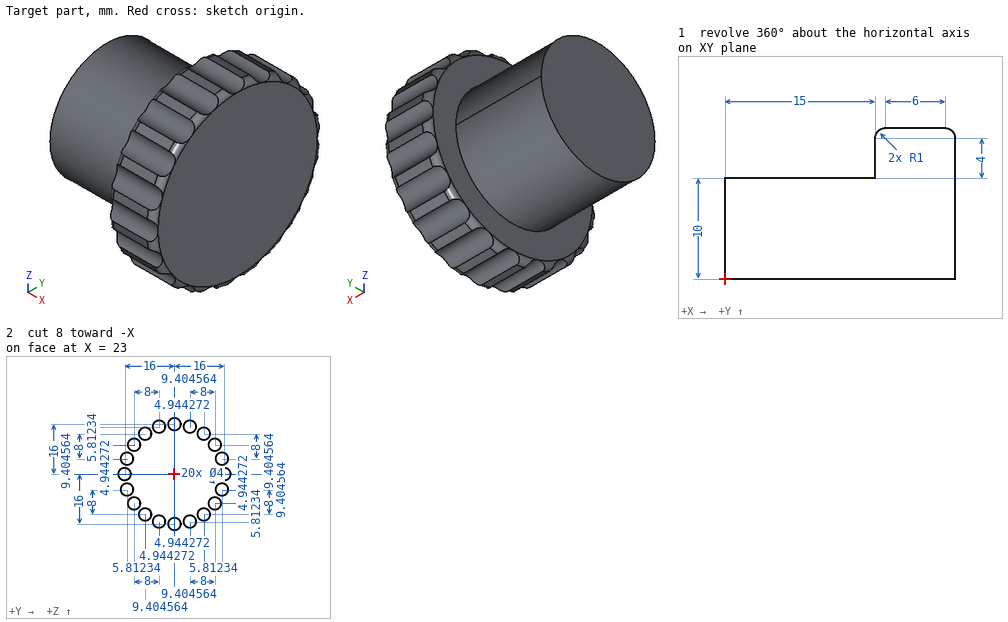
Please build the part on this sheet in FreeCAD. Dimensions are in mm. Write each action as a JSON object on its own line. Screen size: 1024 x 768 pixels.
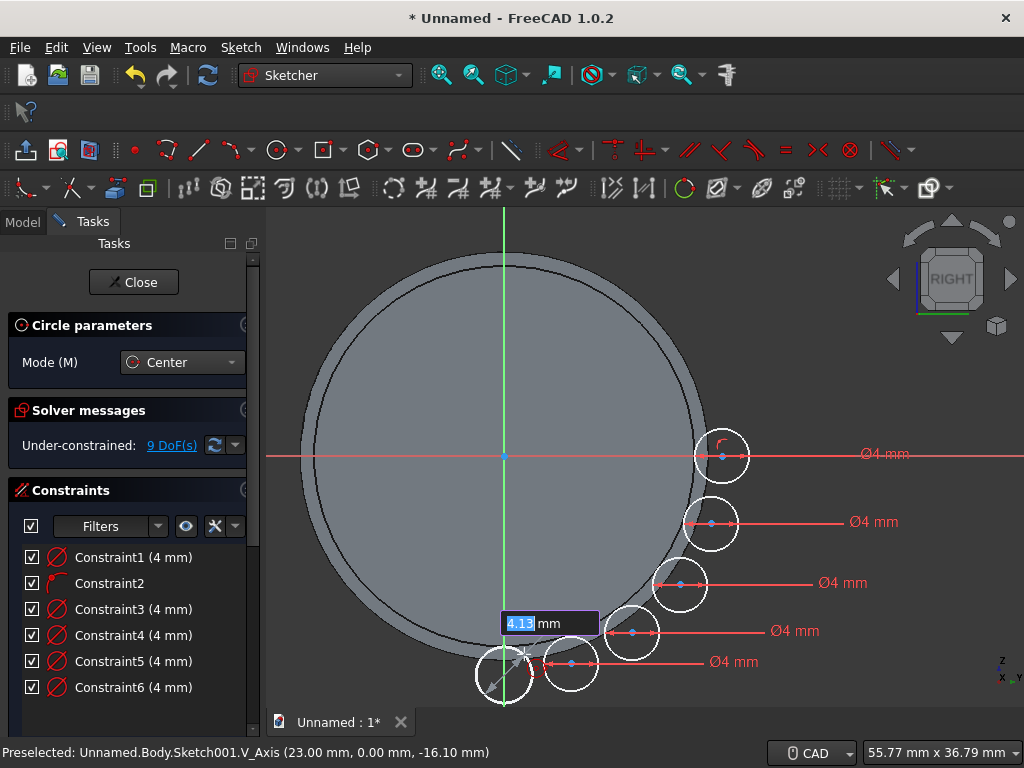
{"action": "type", "text": "4"}
{"action": "key", "text": "Return"}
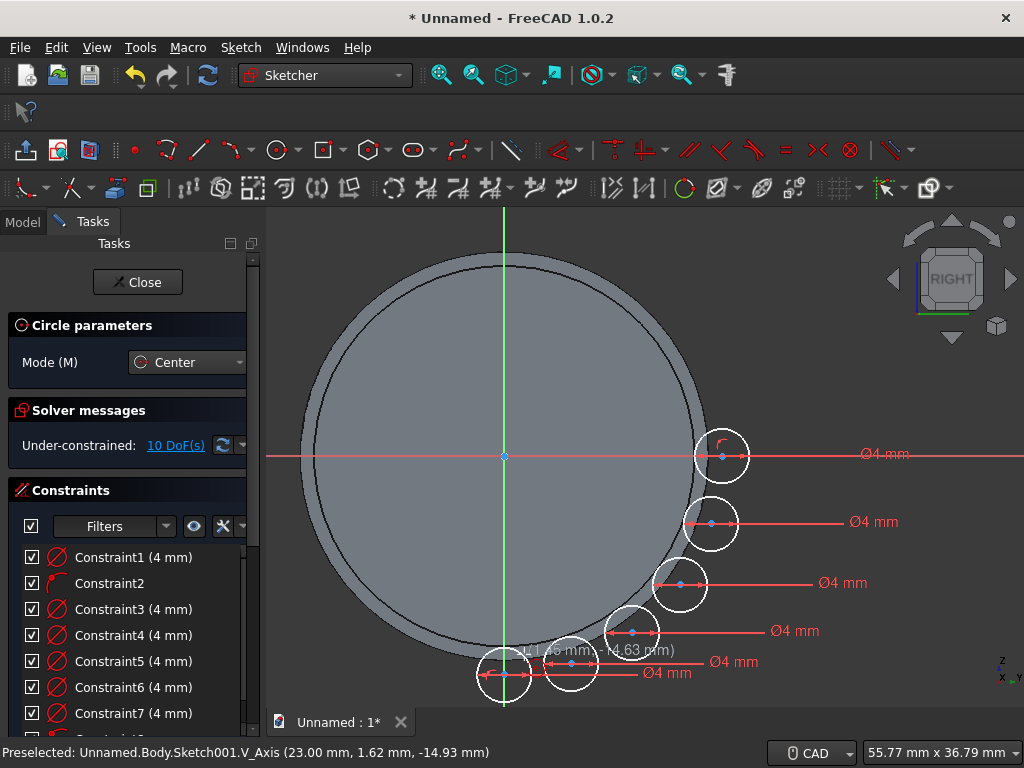
{"action": "left_click", "coordinate": [437, 663]}
{"action": "mouse_move", "coordinate": [456, 644]}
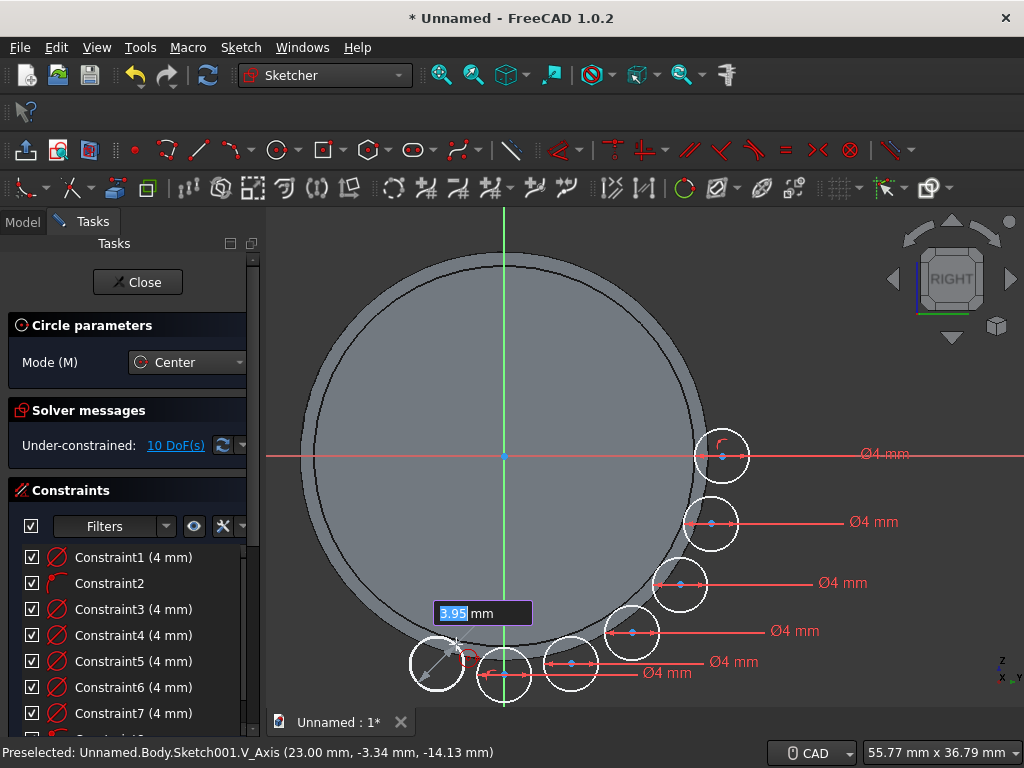
{"action": "type", "text": "4"}
{"action": "key", "text": "Return"}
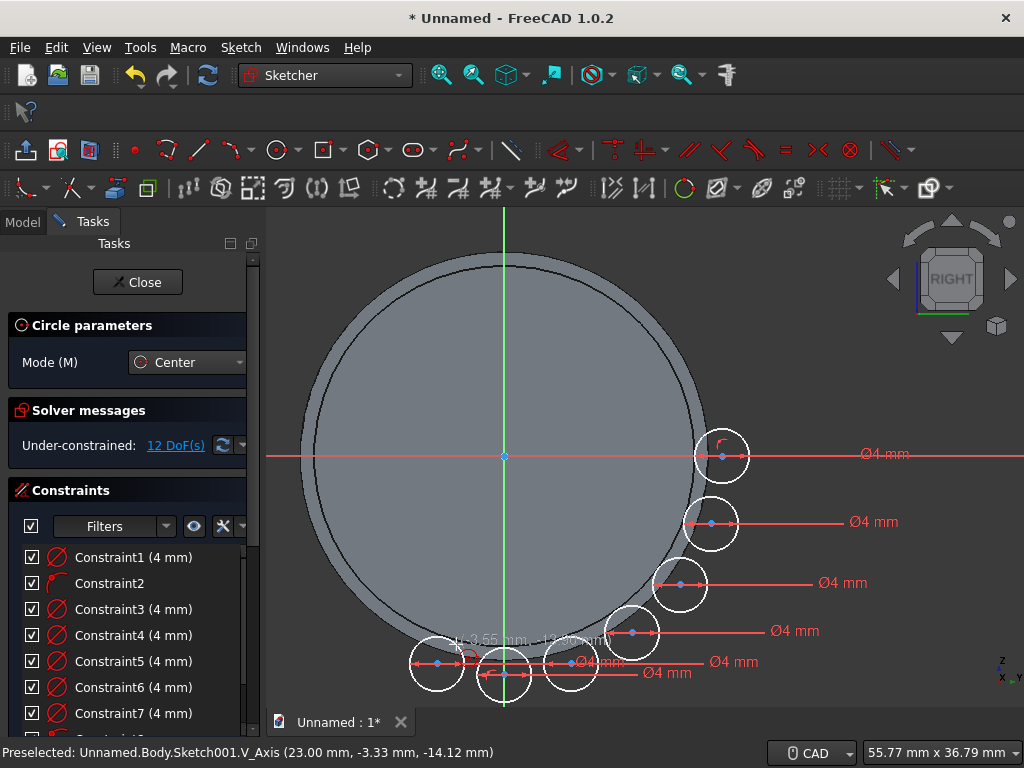
{"action": "left_click", "coordinate": [376, 632]}
{"action": "mouse_move", "coordinate": [396, 613]}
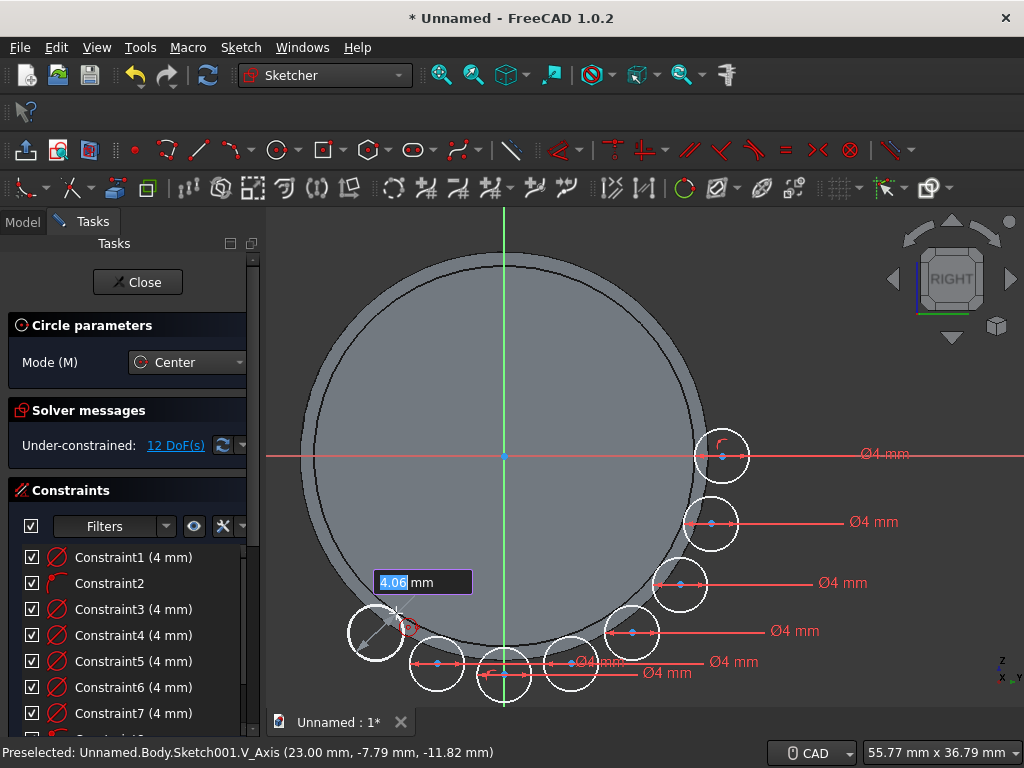
{"action": "type", "text": "4"}
{"action": "key", "text": "Return"}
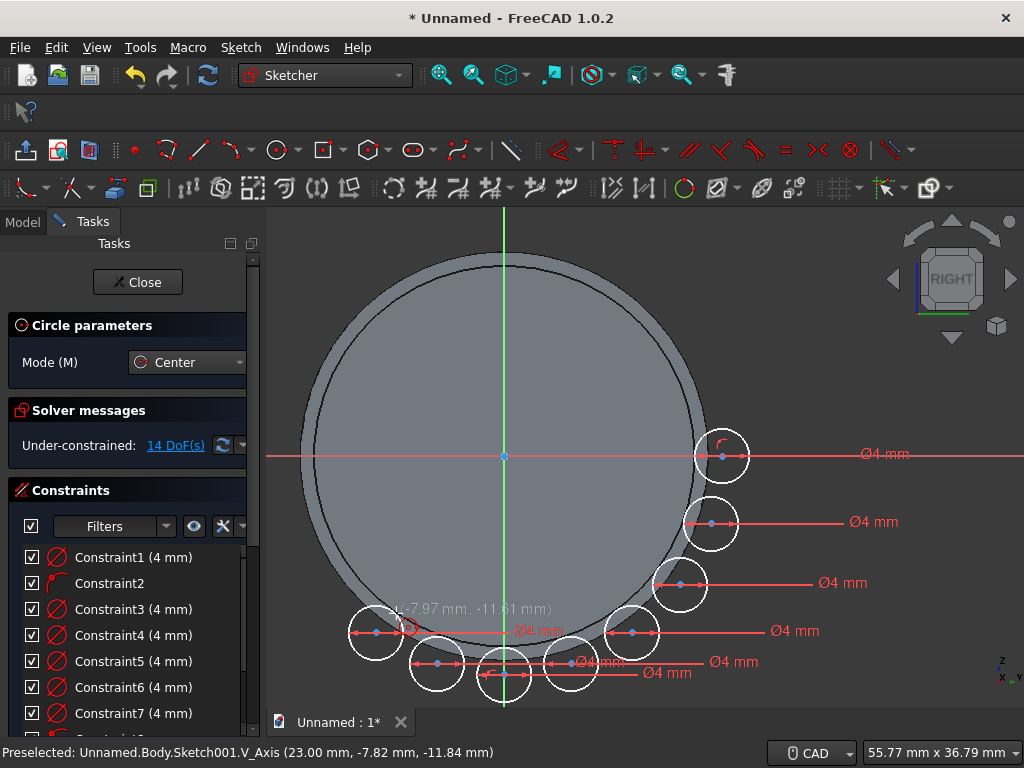
{"action": "left_click", "coordinate": [328, 584]}
{"action": "mouse_move", "coordinate": [348, 565]}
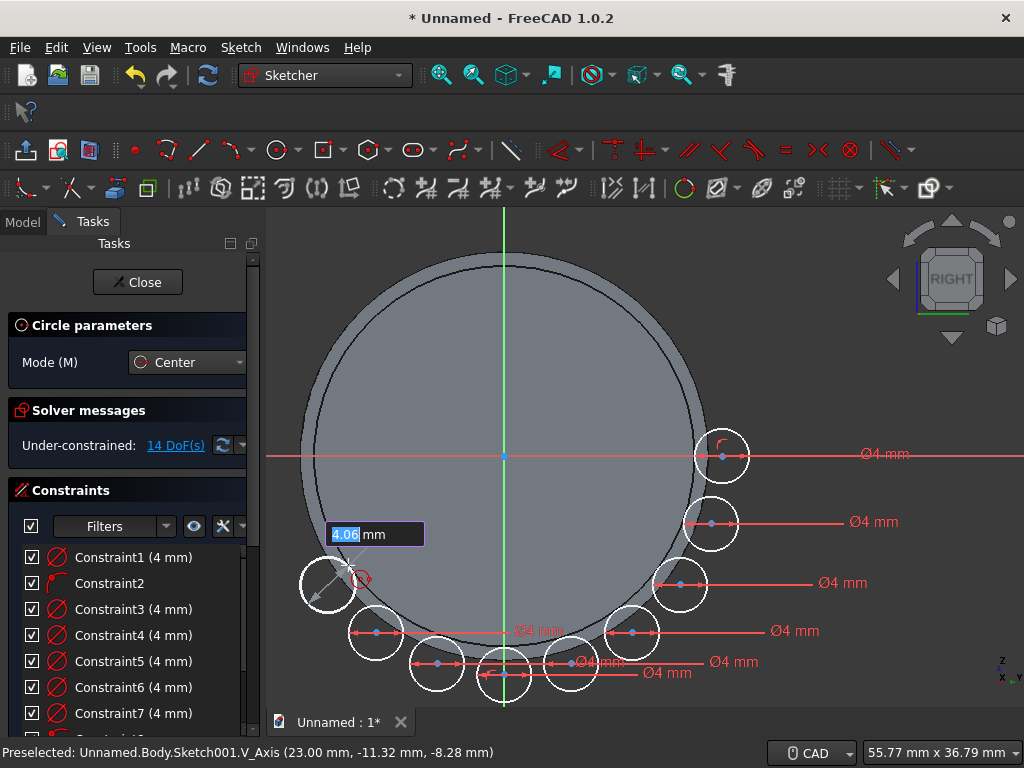
{"action": "type", "text": "4"}
{"action": "key", "text": "Return"}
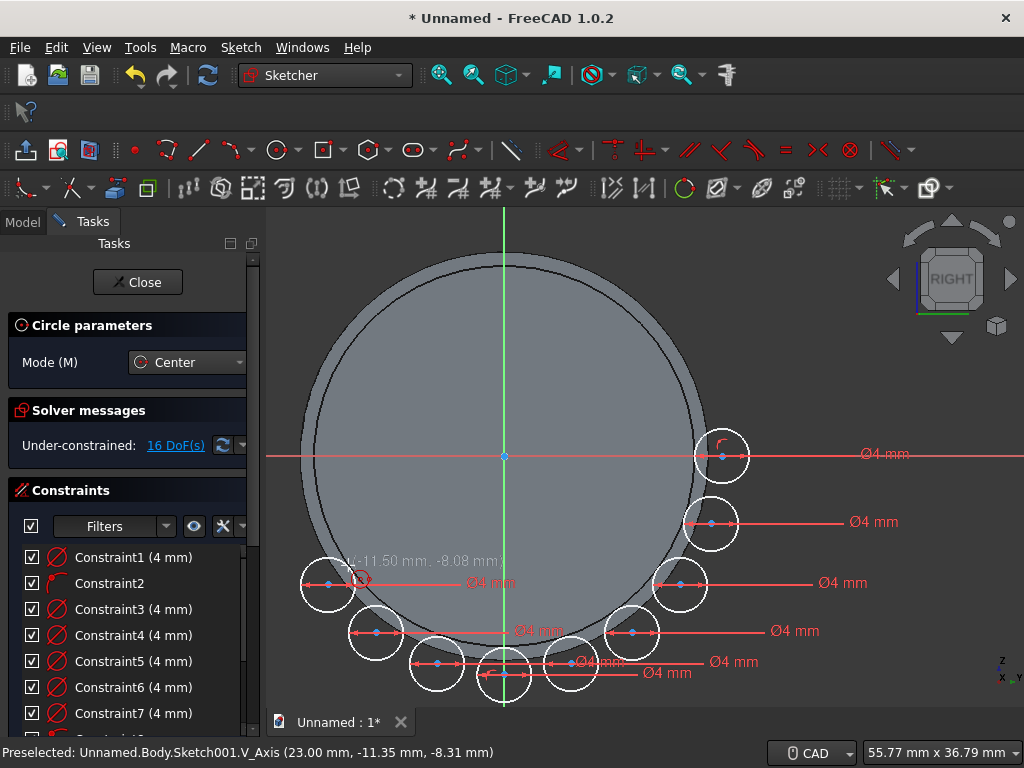
{"action": "left_click", "coordinate": [297, 523]}
{"action": "mouse_move", "coordinate": [317, 504]}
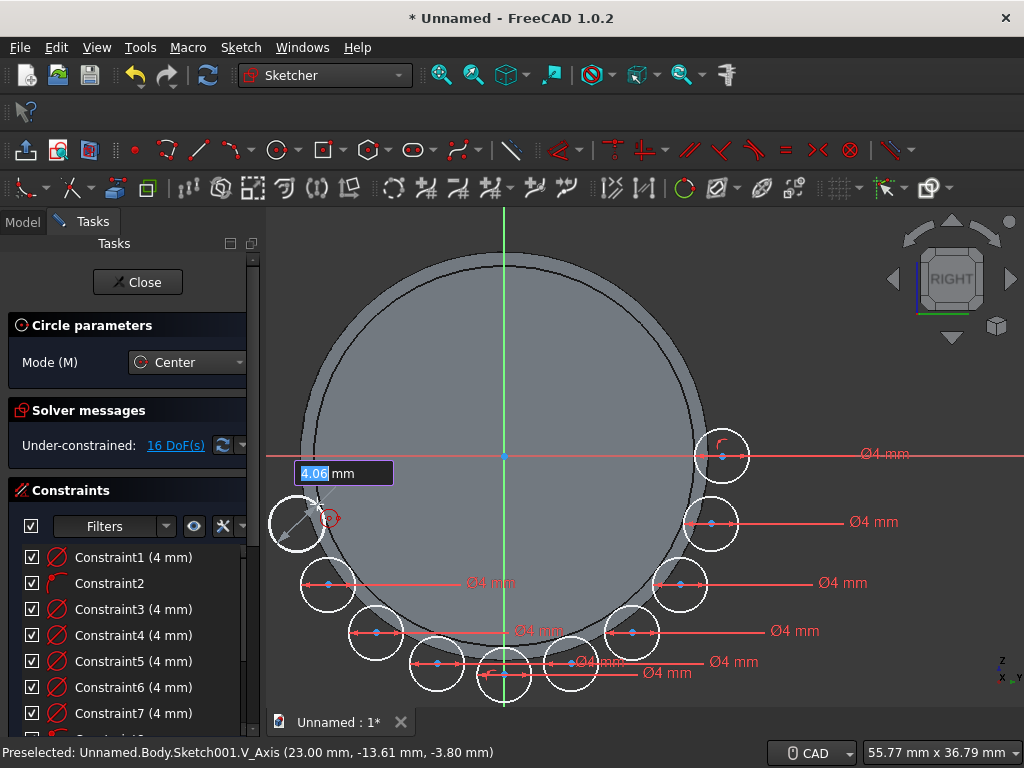
{"action": "type", "text": "4"}
{"action": "key", "text": "Return"}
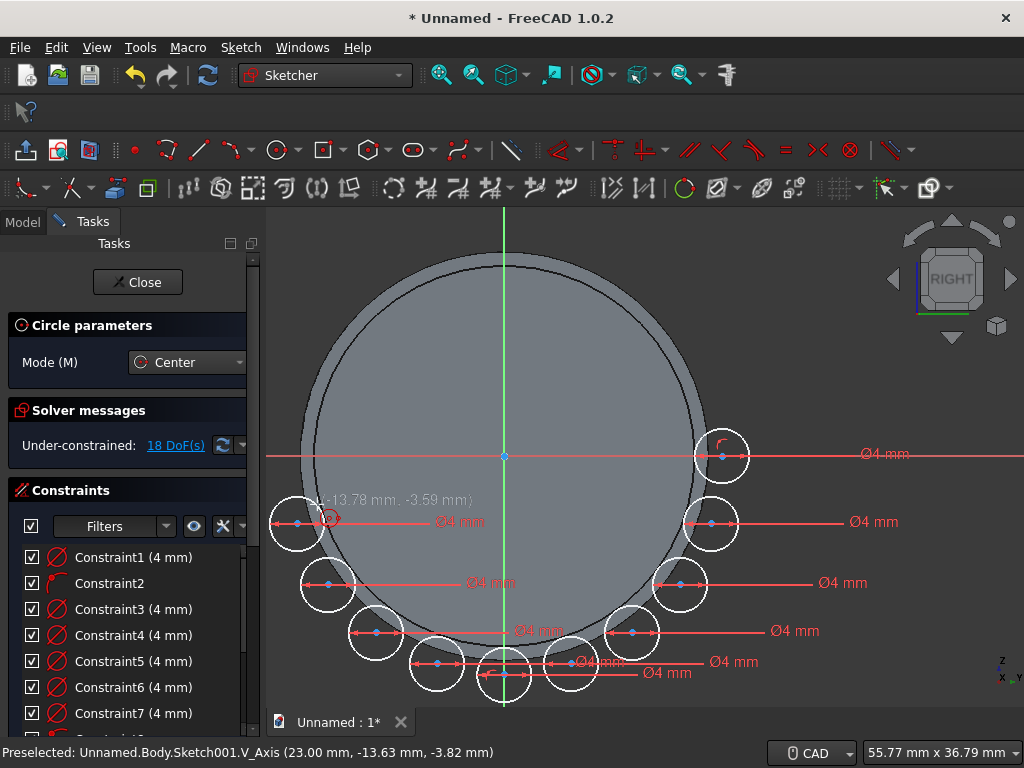
{"action": "scroll", "coordinate": [723, 459], "scroll_direction": "down", "scroll_amount": 2}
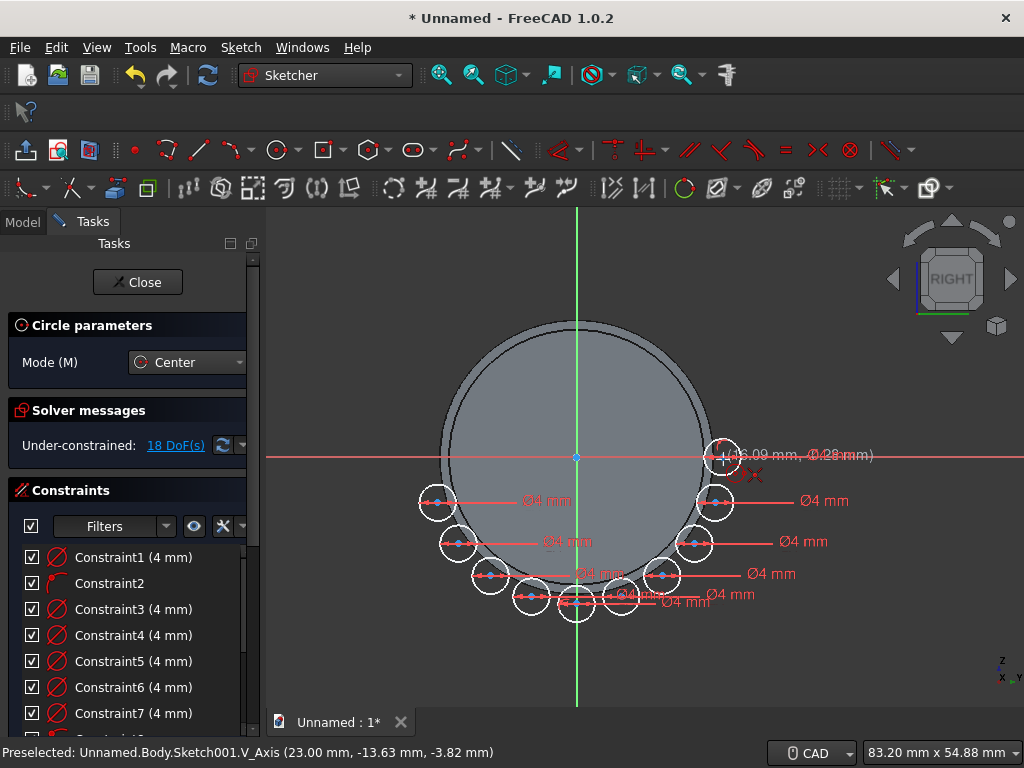
{"action": "scroll", "coordinate": [431, 457], "scroll_direction": "up", "scroll_amount": 2}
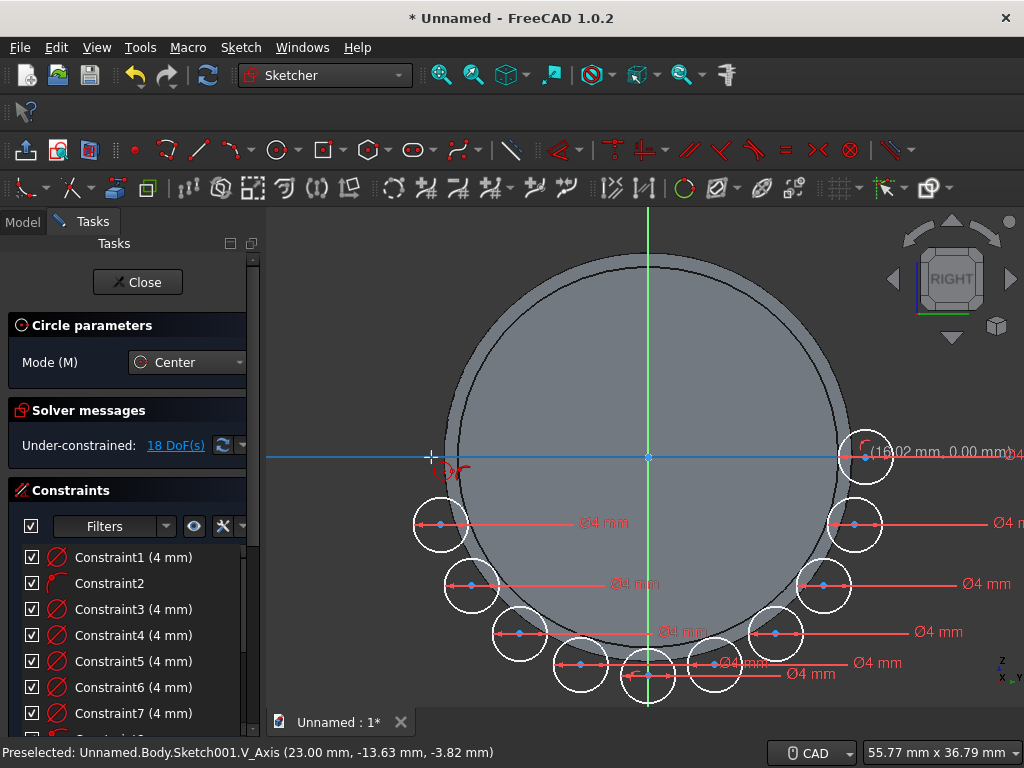
{"action": "left_click", "coordinate": [431, 457]}
{"action": "mouse_move", "coordinate": [450, 438]}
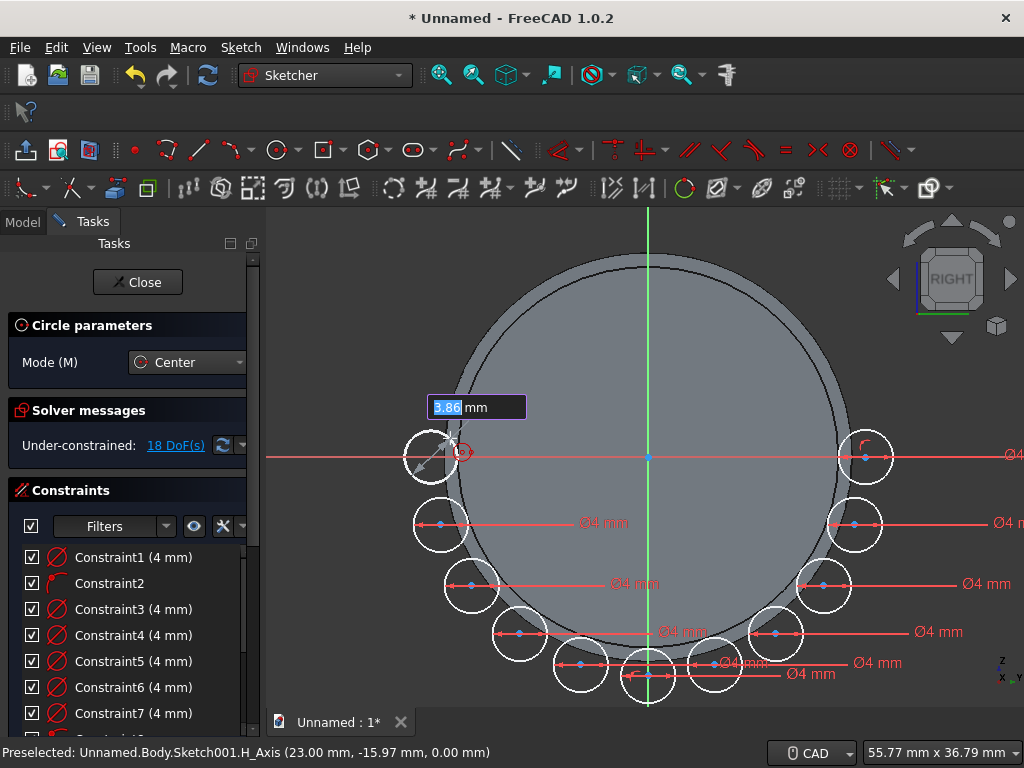
{"action": "type", "text": "4"}
{"action": "key", "text": "Return"}